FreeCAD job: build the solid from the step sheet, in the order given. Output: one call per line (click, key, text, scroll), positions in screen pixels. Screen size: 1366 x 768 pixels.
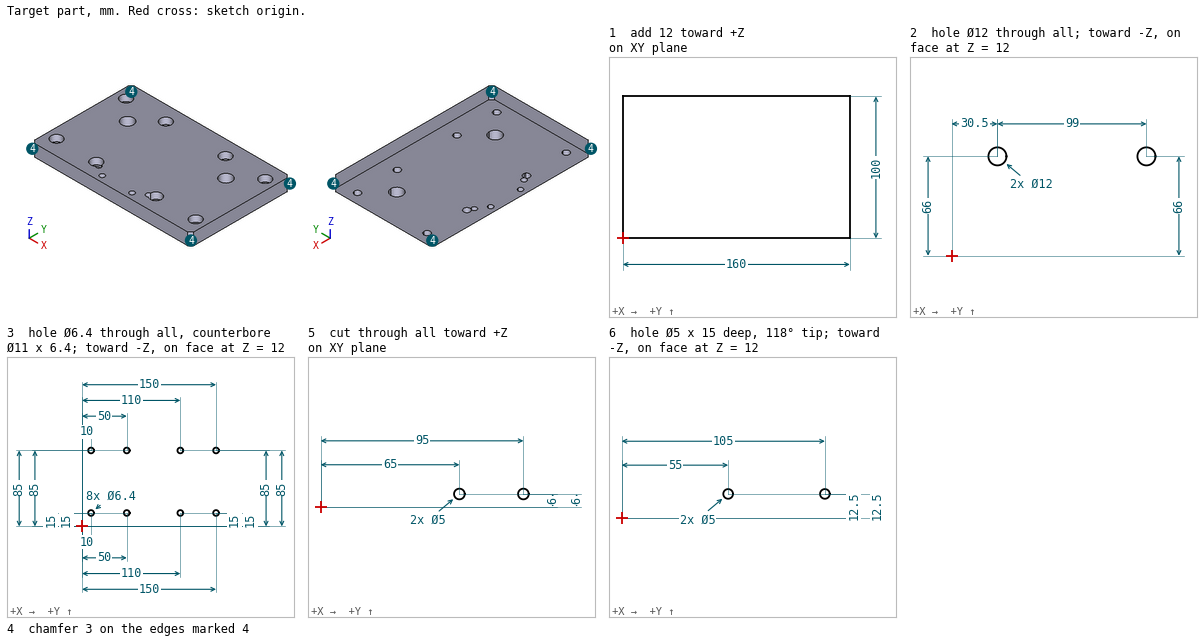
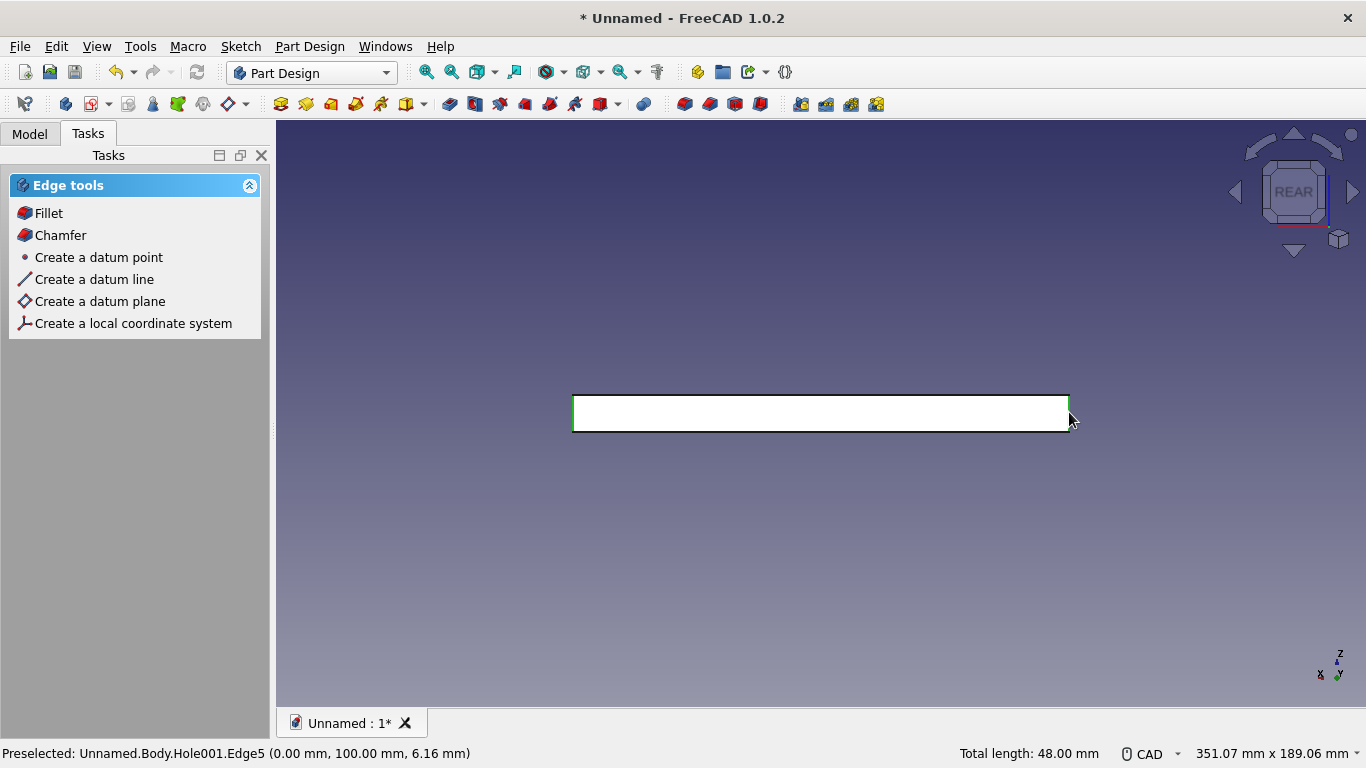
click(710, 104)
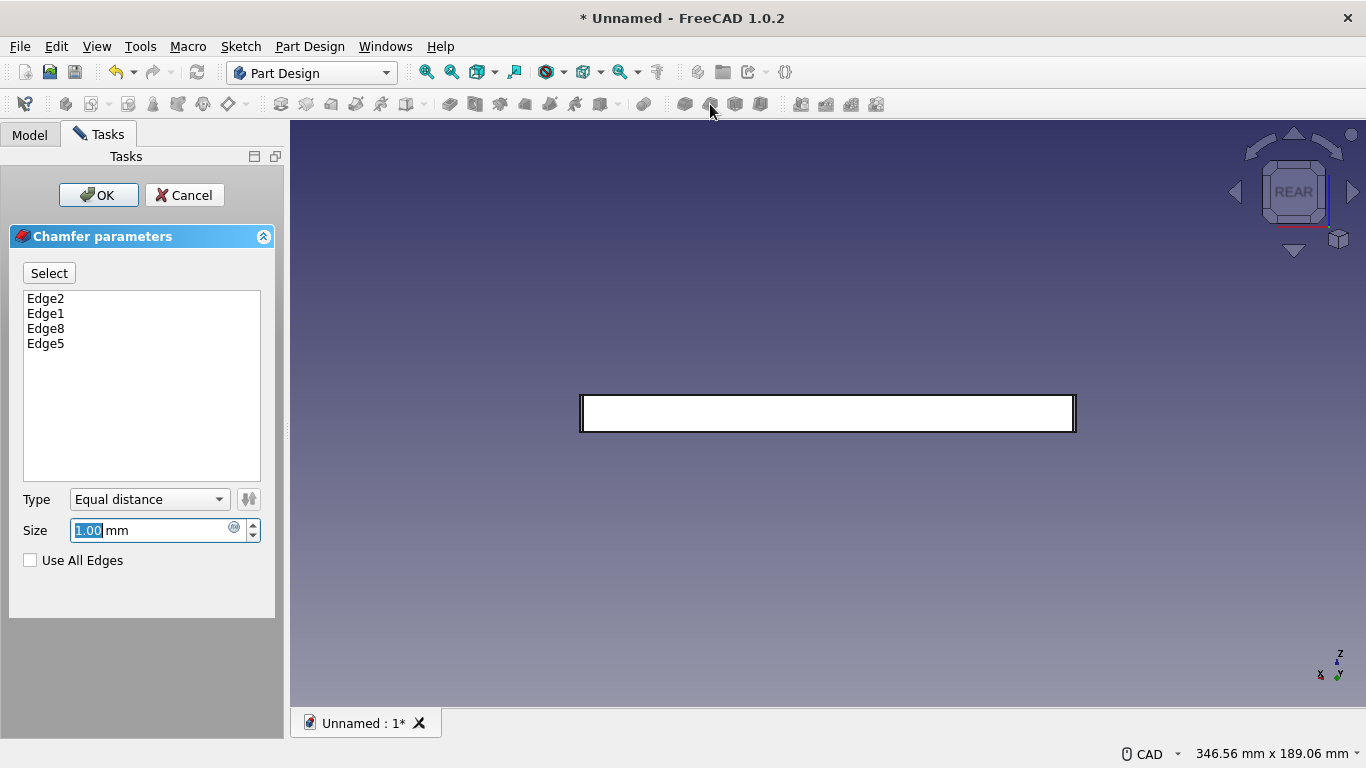
text(3)
key(Tab)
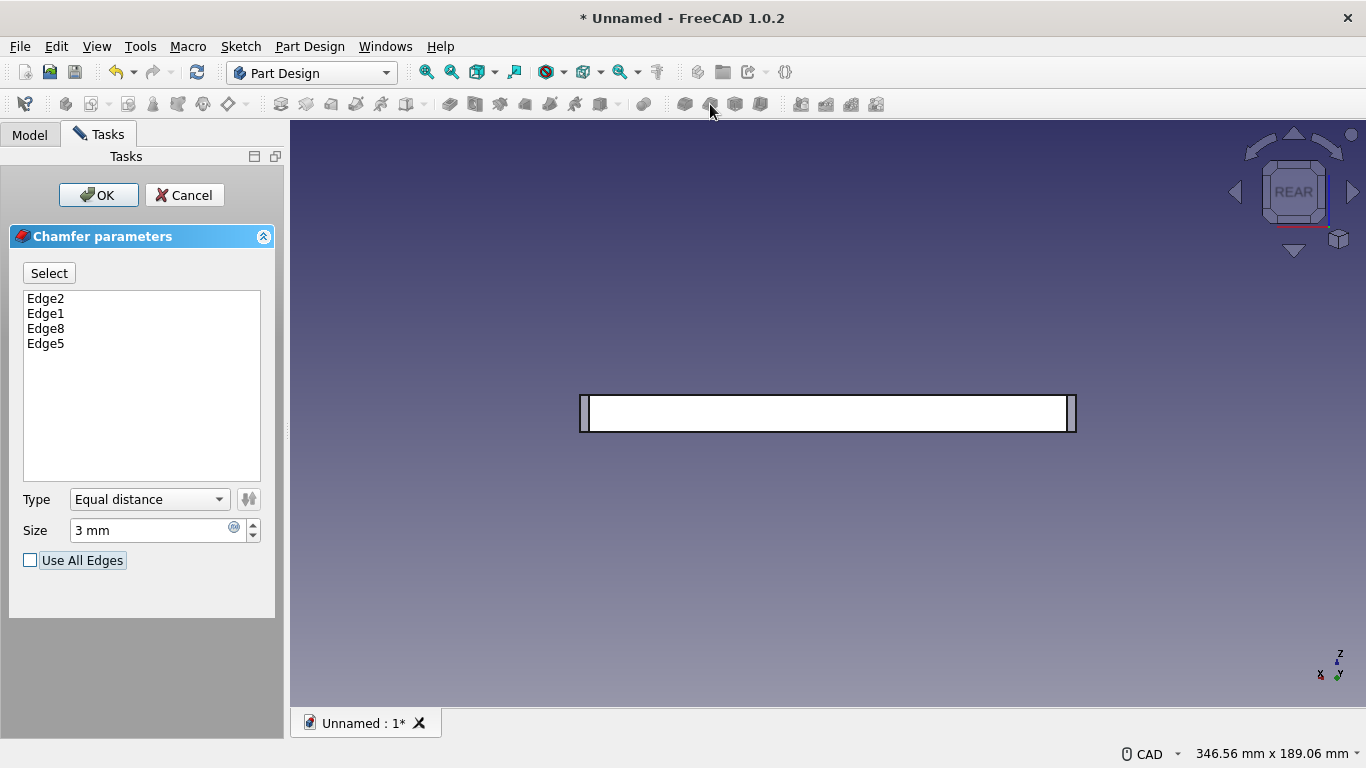
click(99, 195)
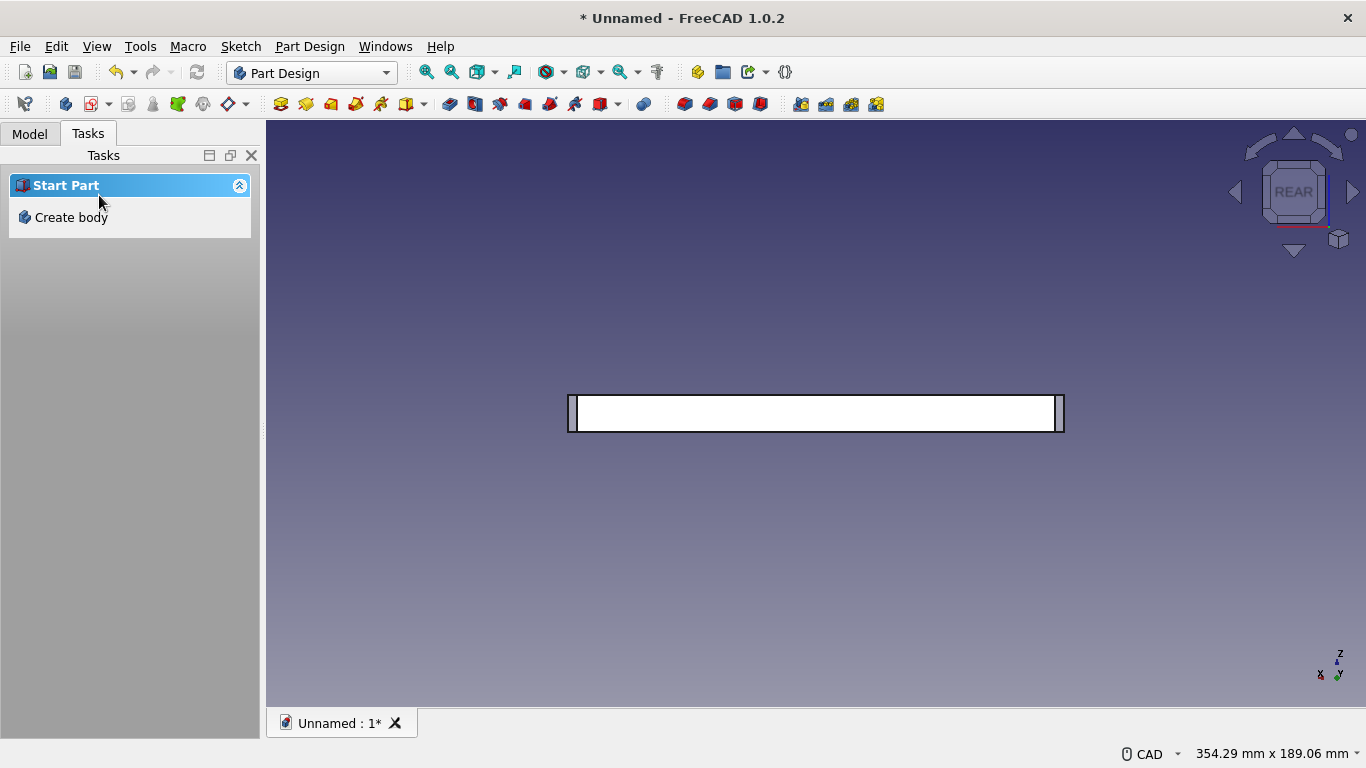
click(90, 104)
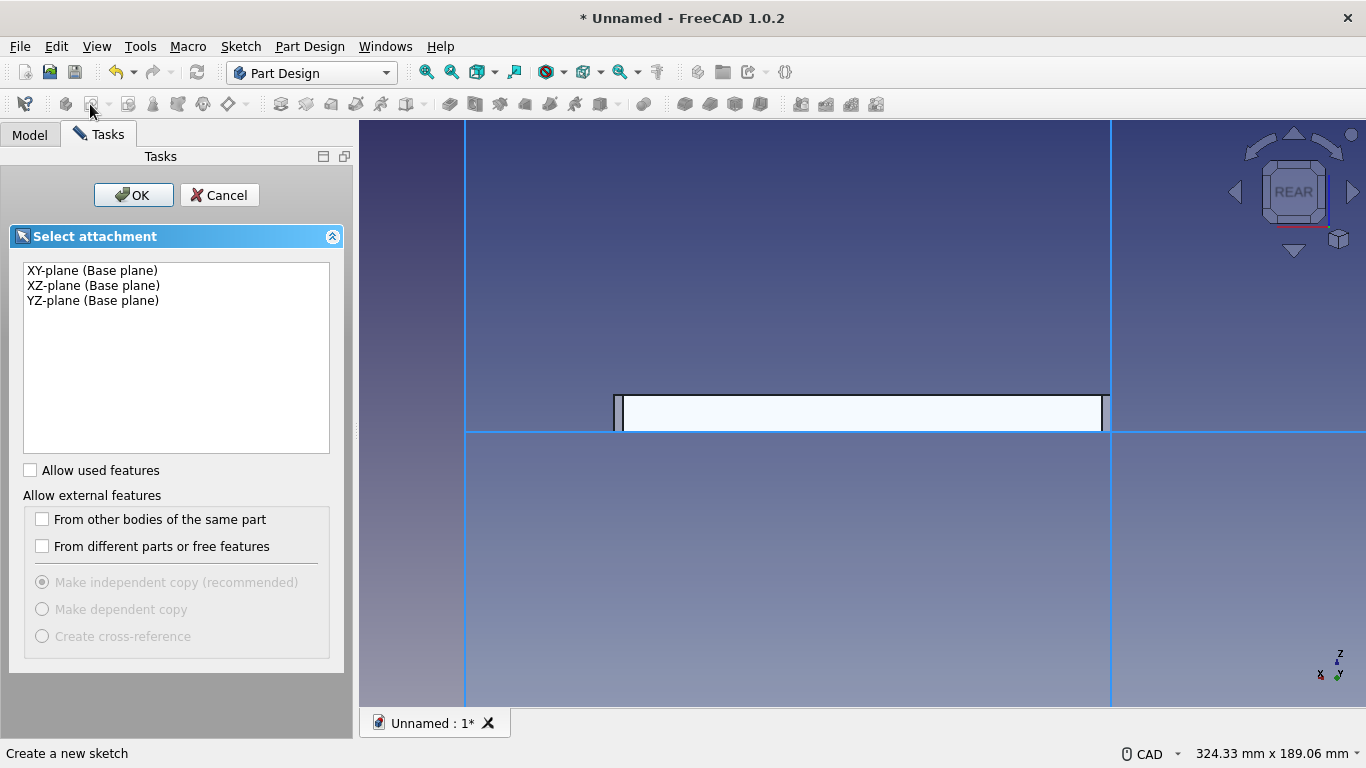
click(84, 270)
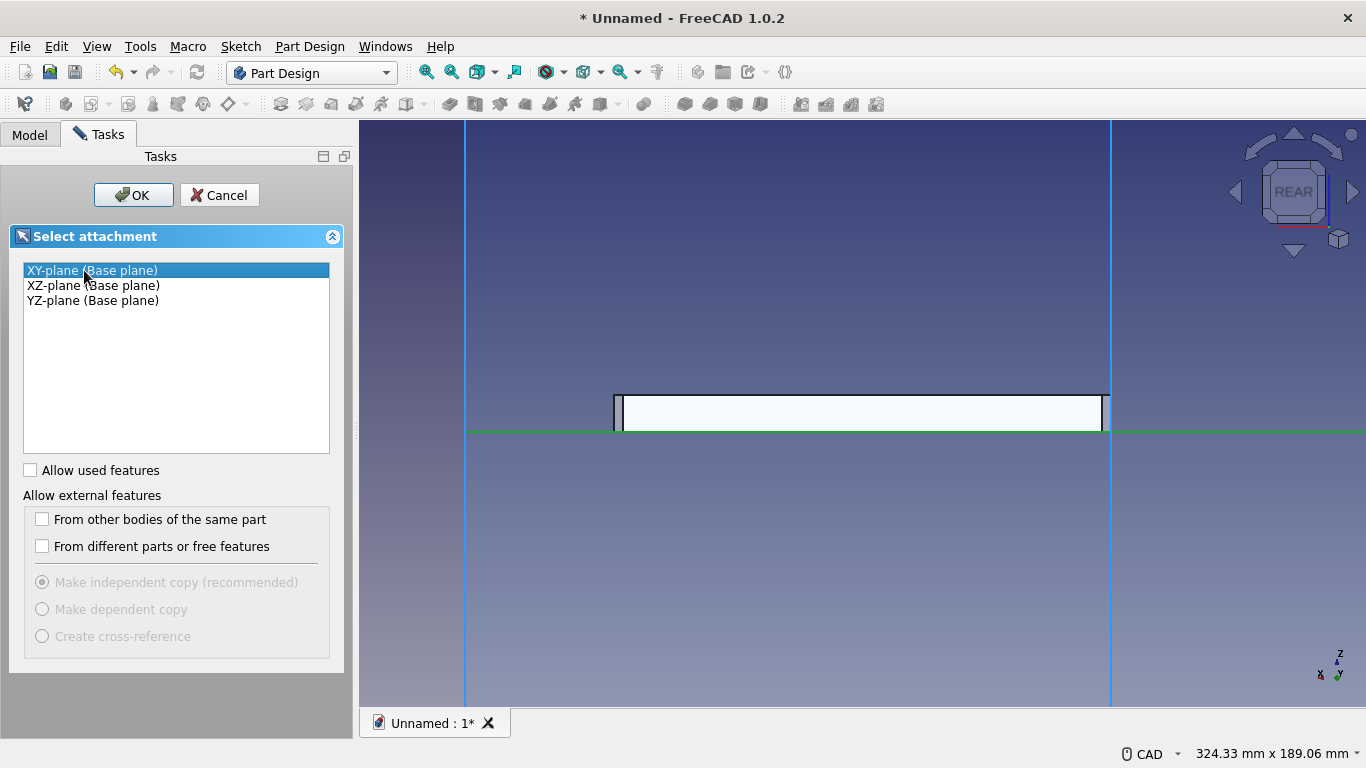
click(134, 195)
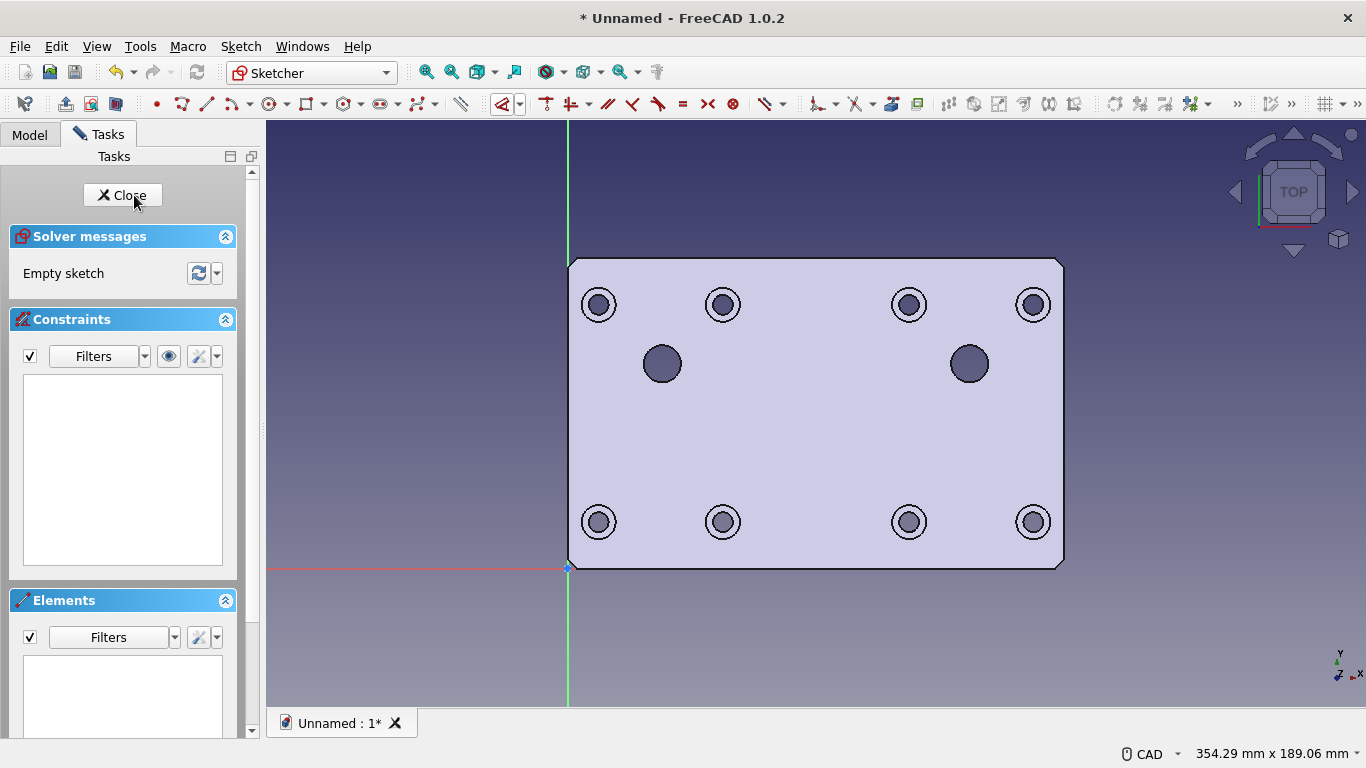
key(q)
key(s)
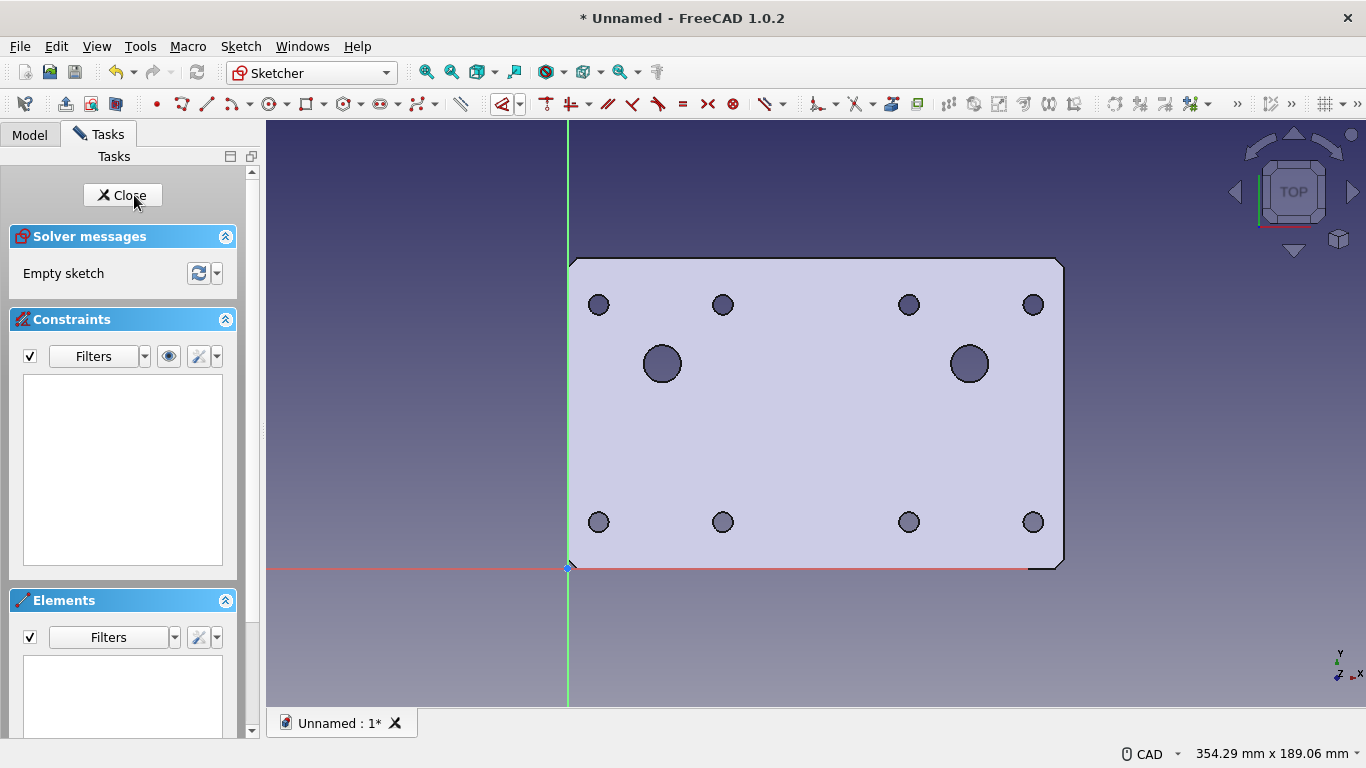
scroll(830, 577, up, 9)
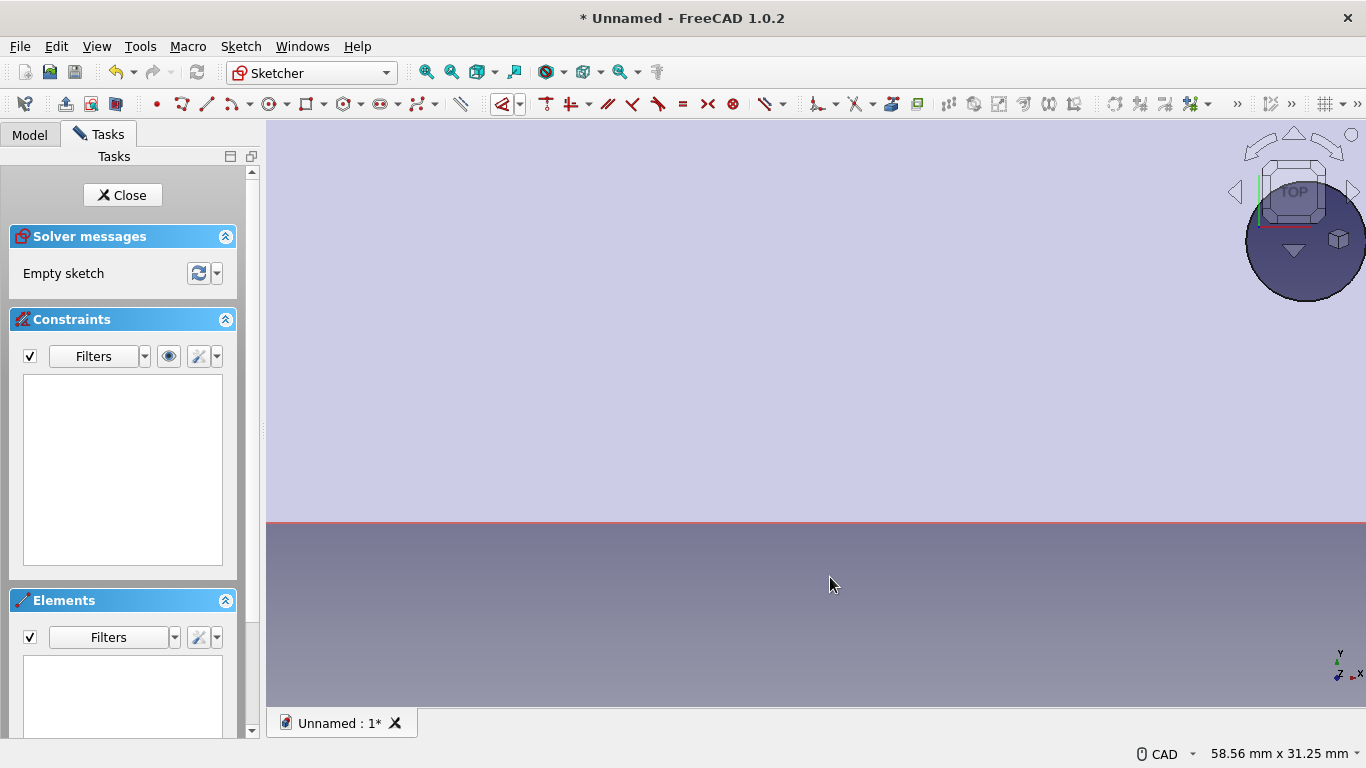
key(g)
key(c)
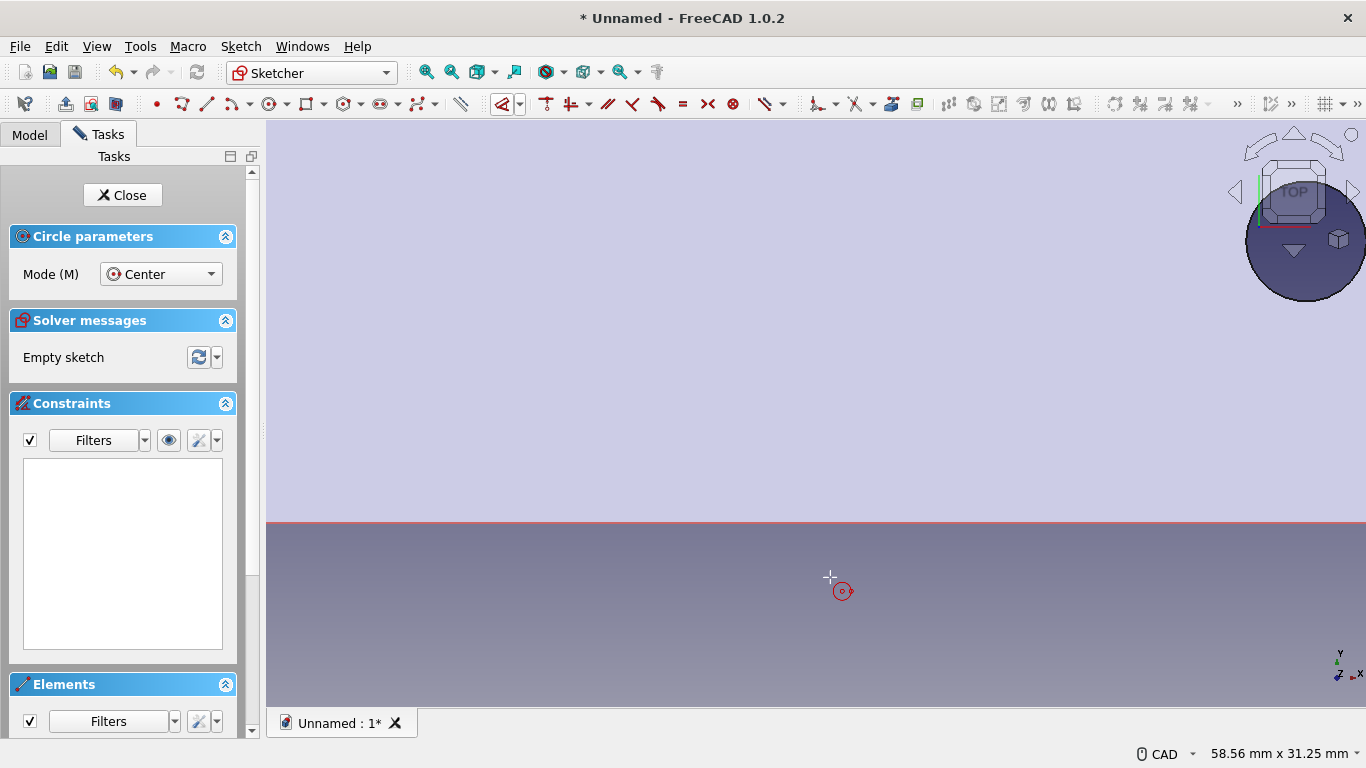
click(461, 410)
click(494, 377)